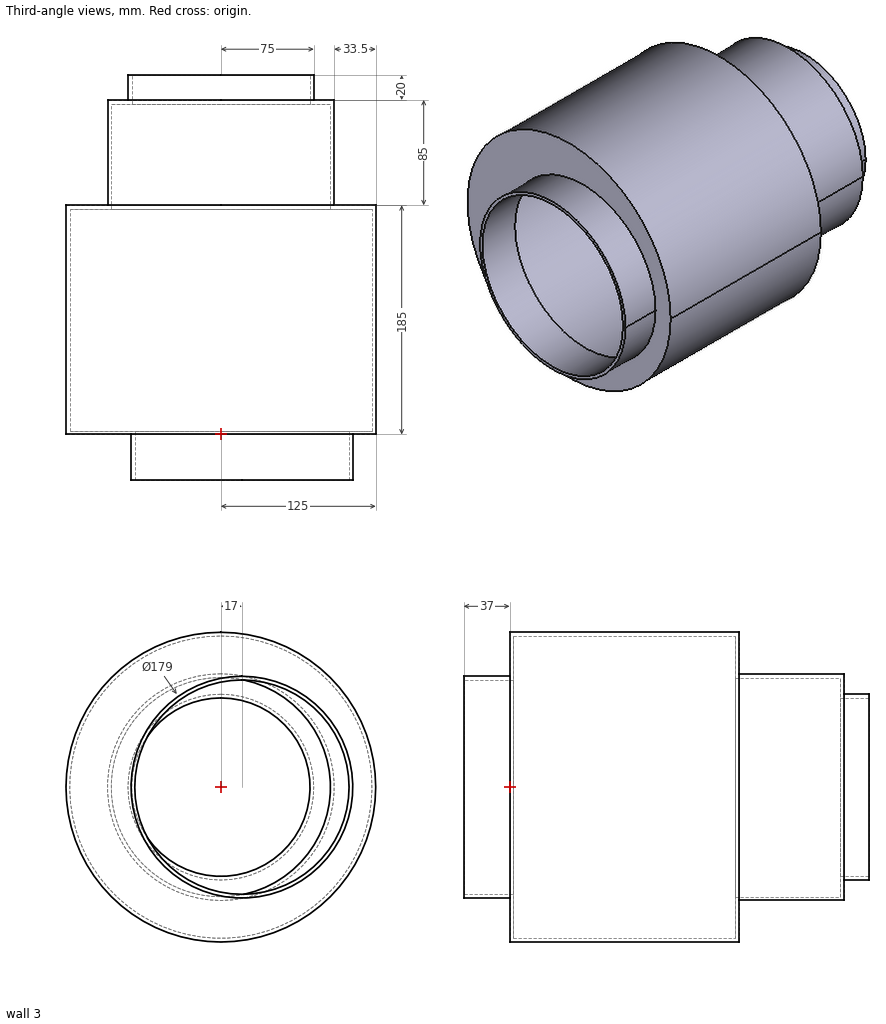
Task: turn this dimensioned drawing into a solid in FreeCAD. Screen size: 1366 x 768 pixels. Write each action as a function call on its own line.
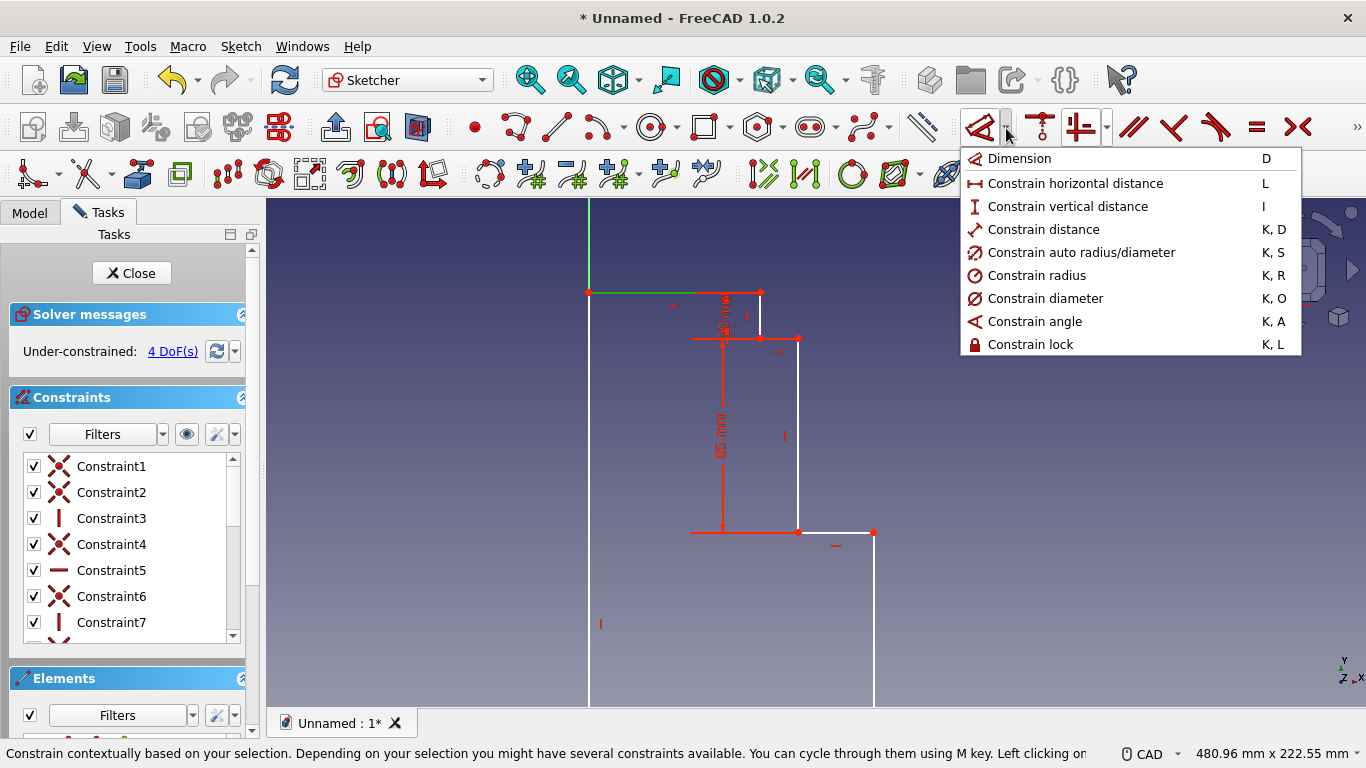
click(1131, 184)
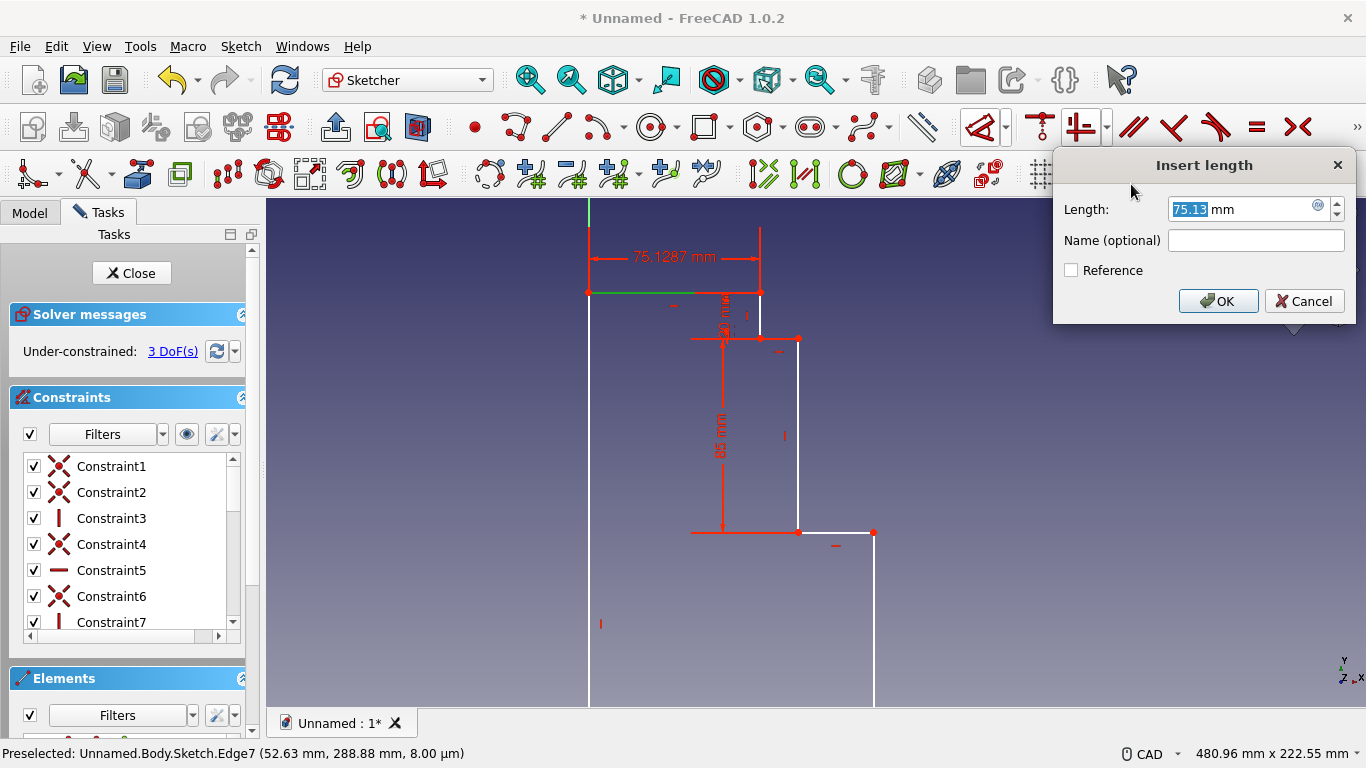
text(75)
key(Return)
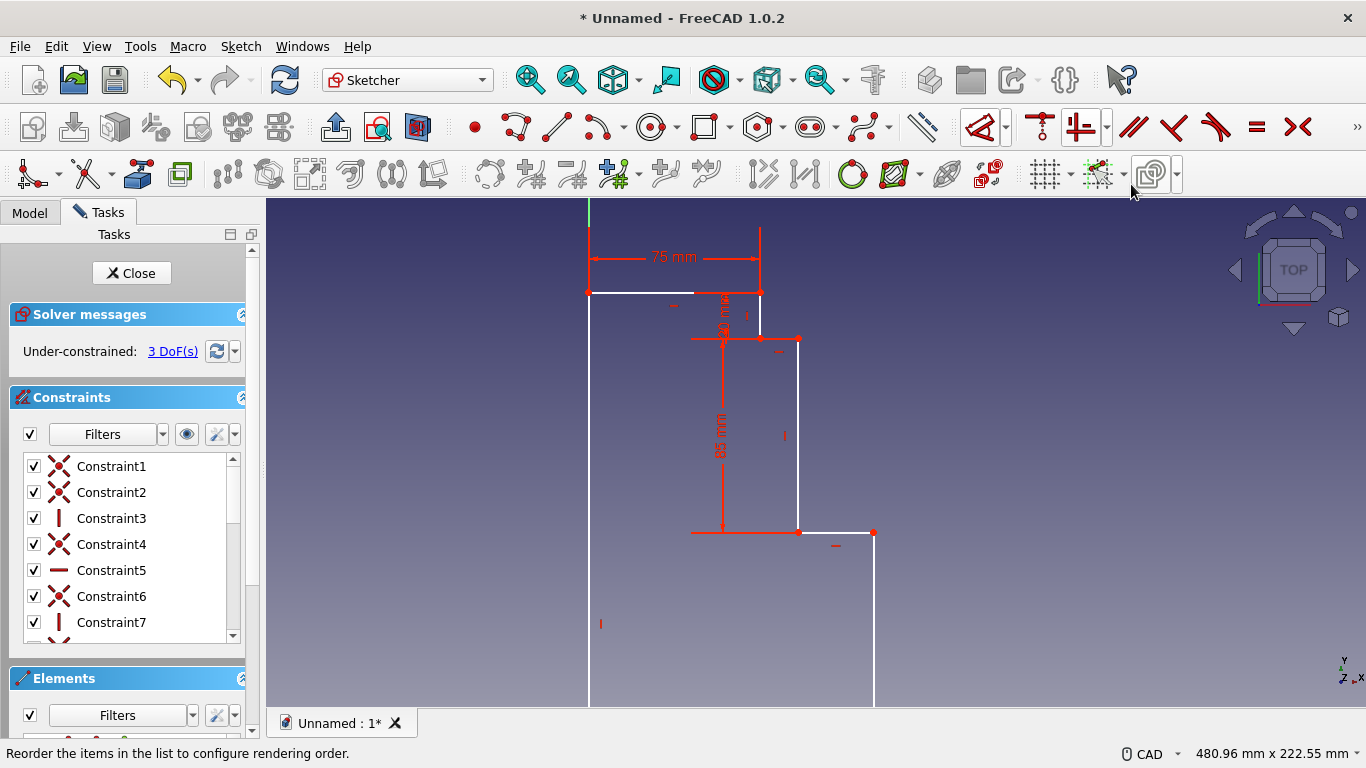
scroll(761, 314, down, 4)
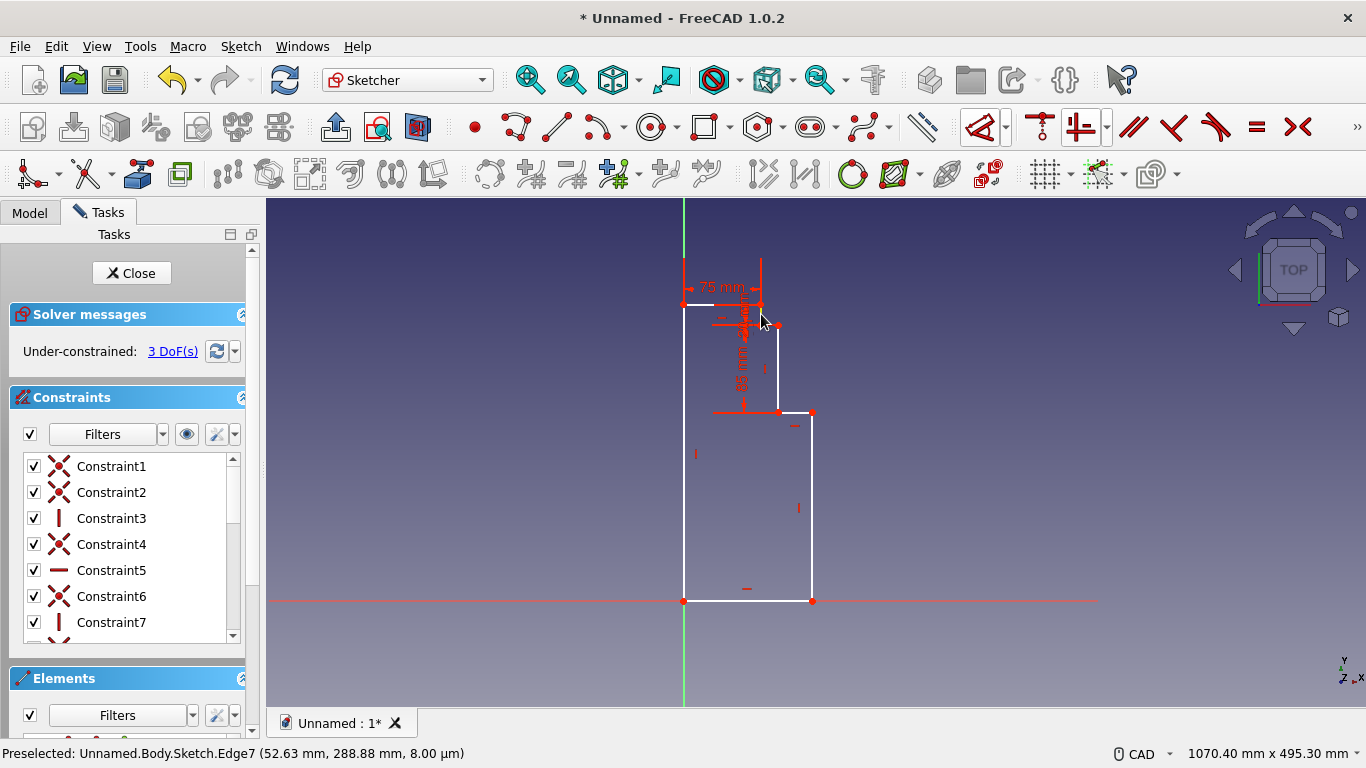
click(722, 601)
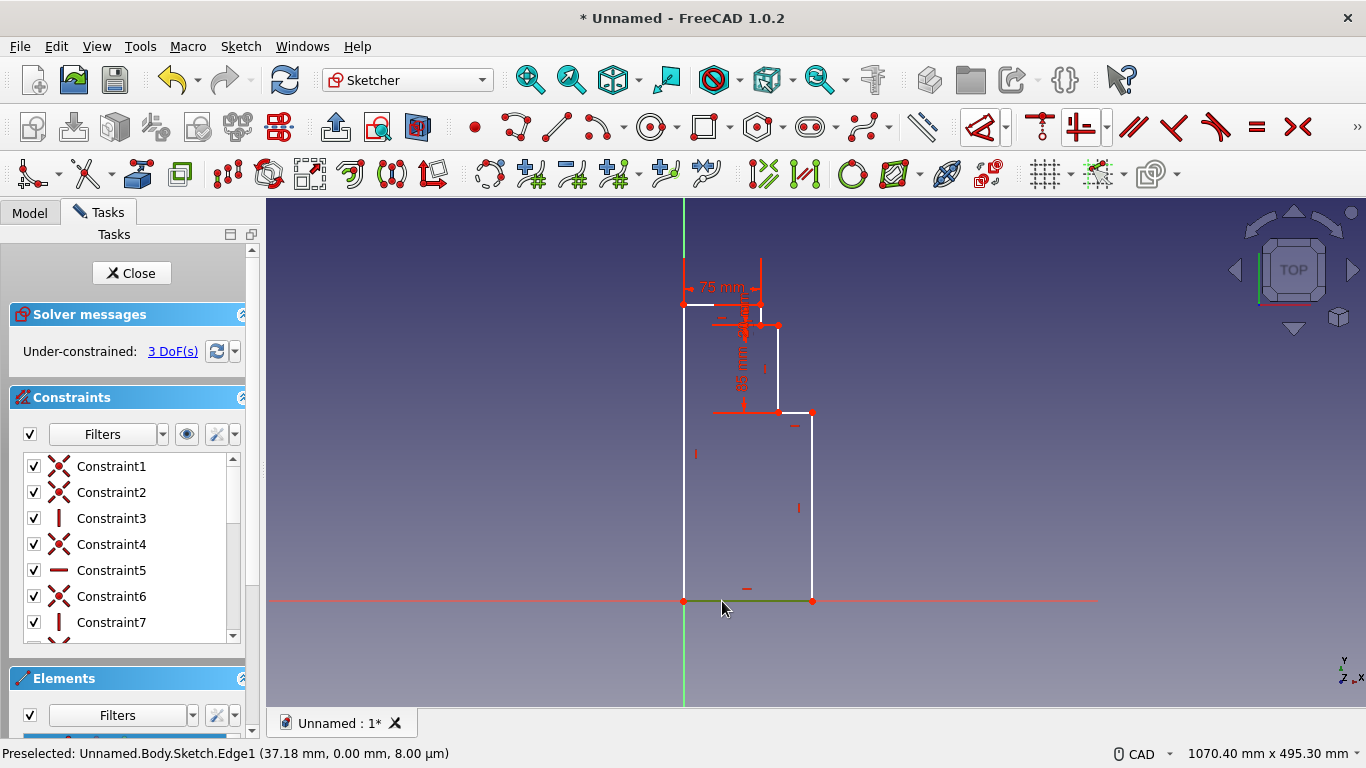
click(1006, 128)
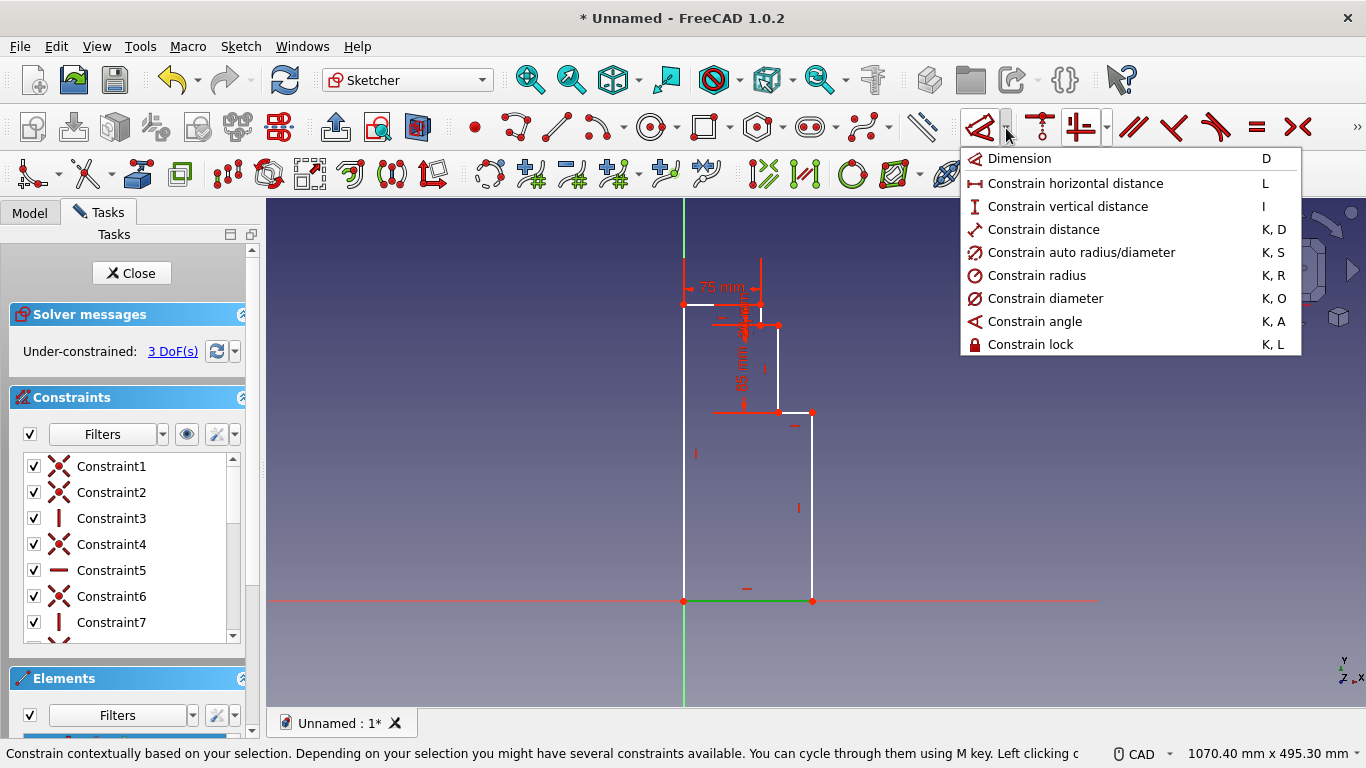
click(1131, 184)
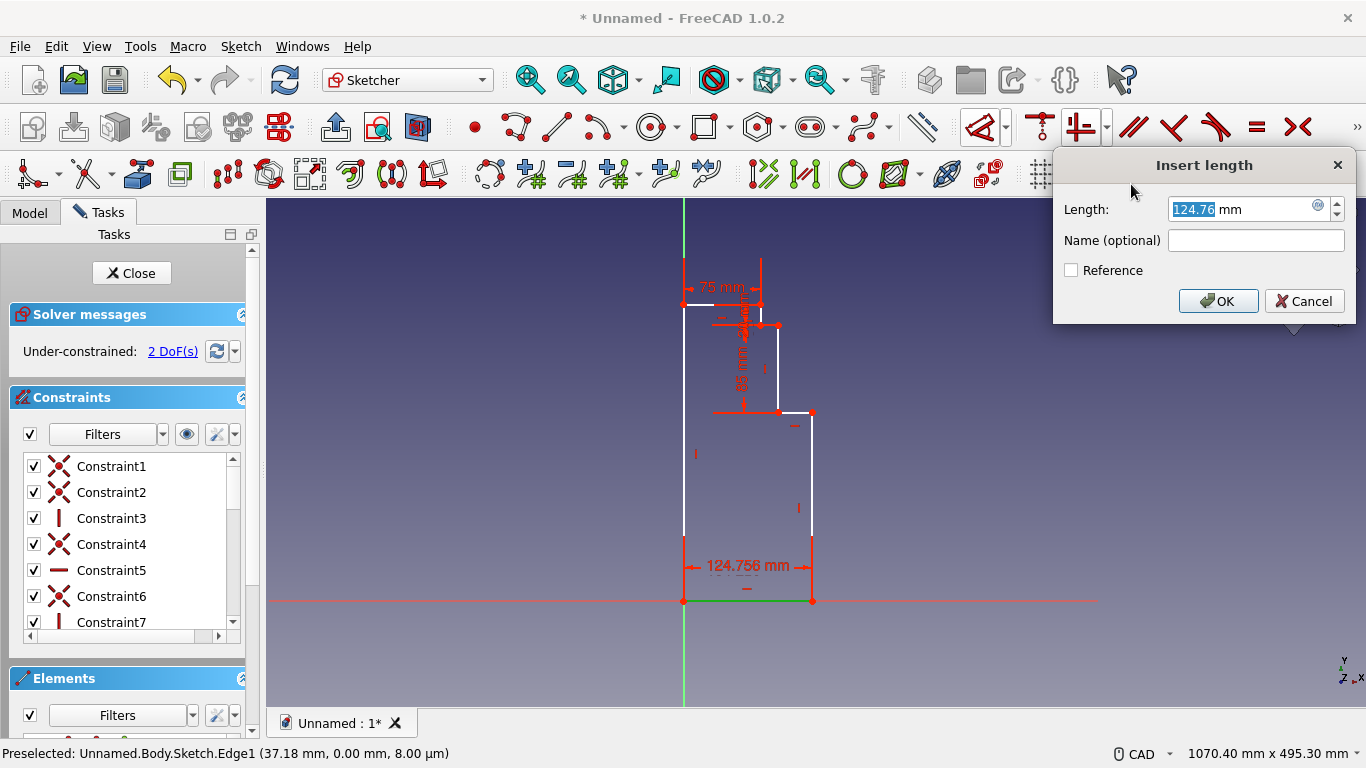
text(125)
key(Return)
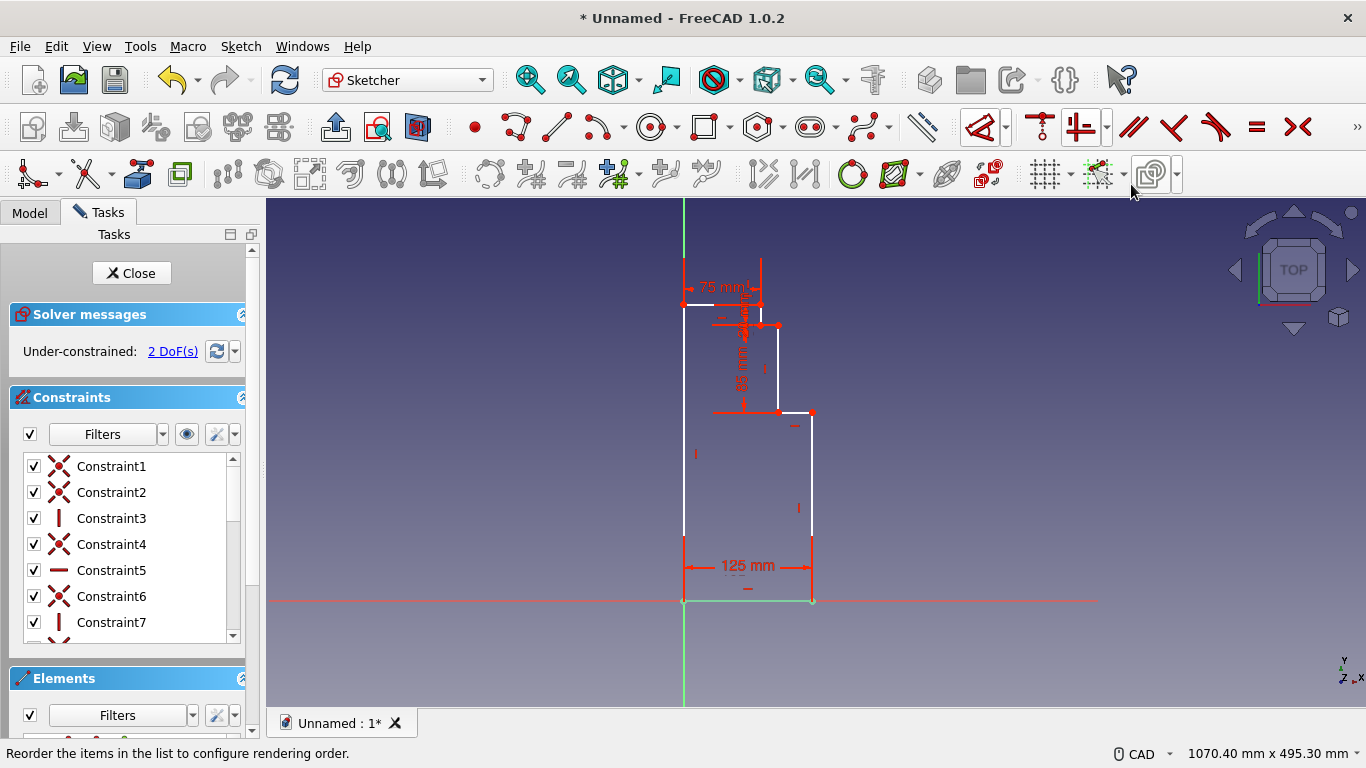
click(812, 545)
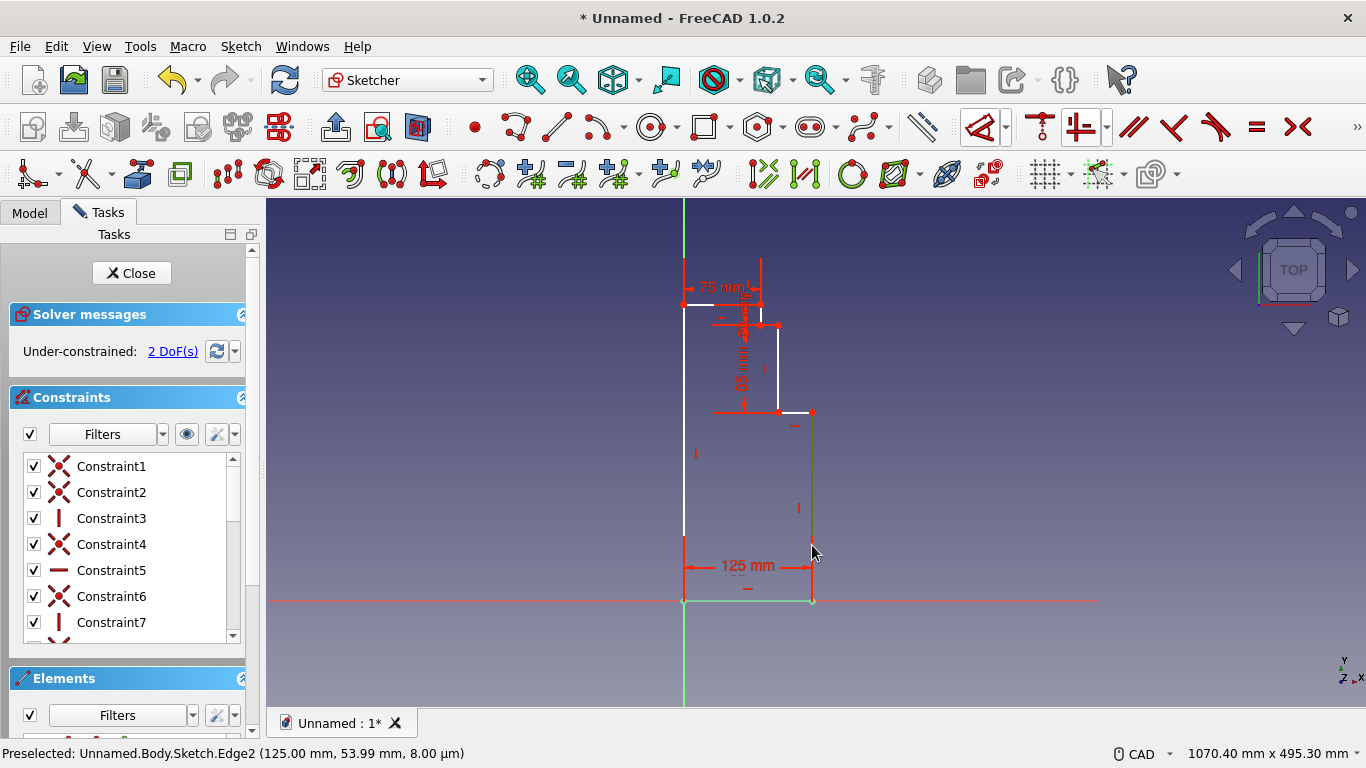
click(1006, 128)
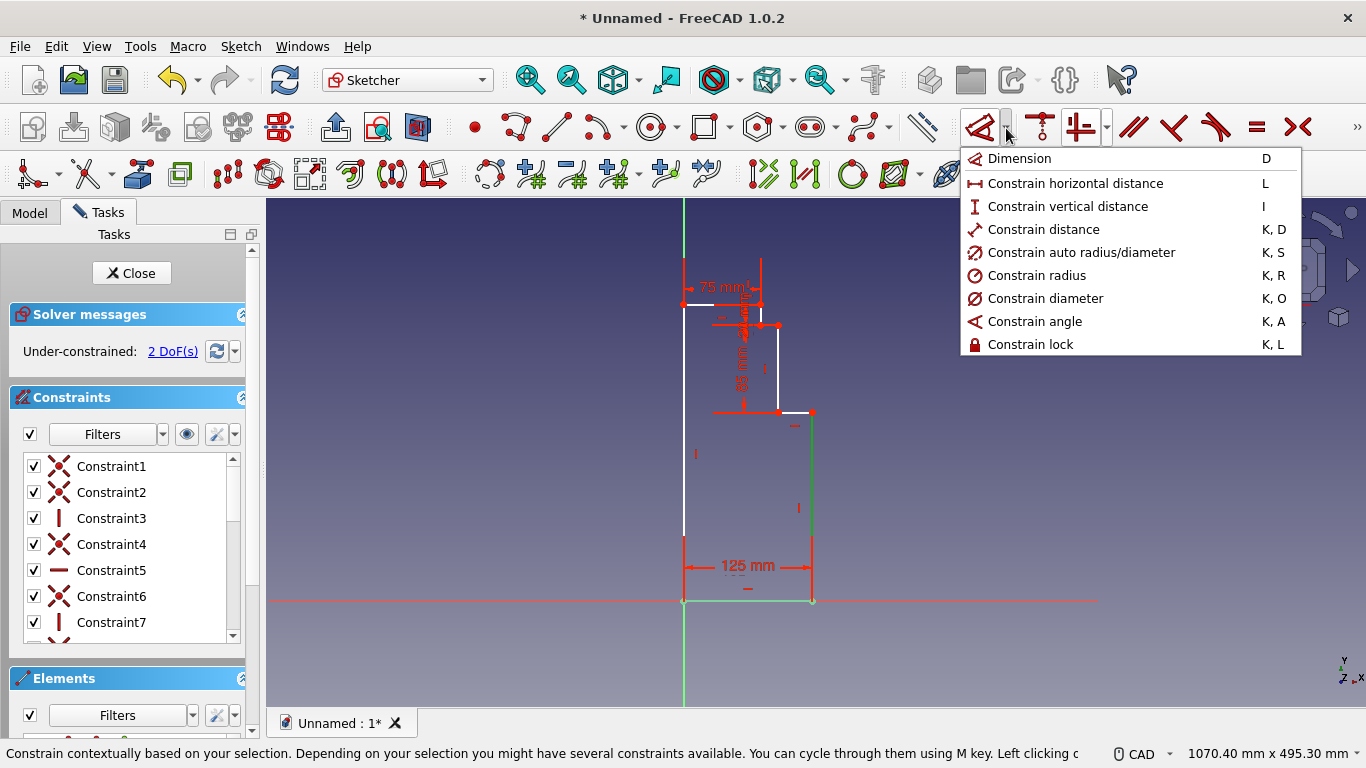
click(1131, 206)